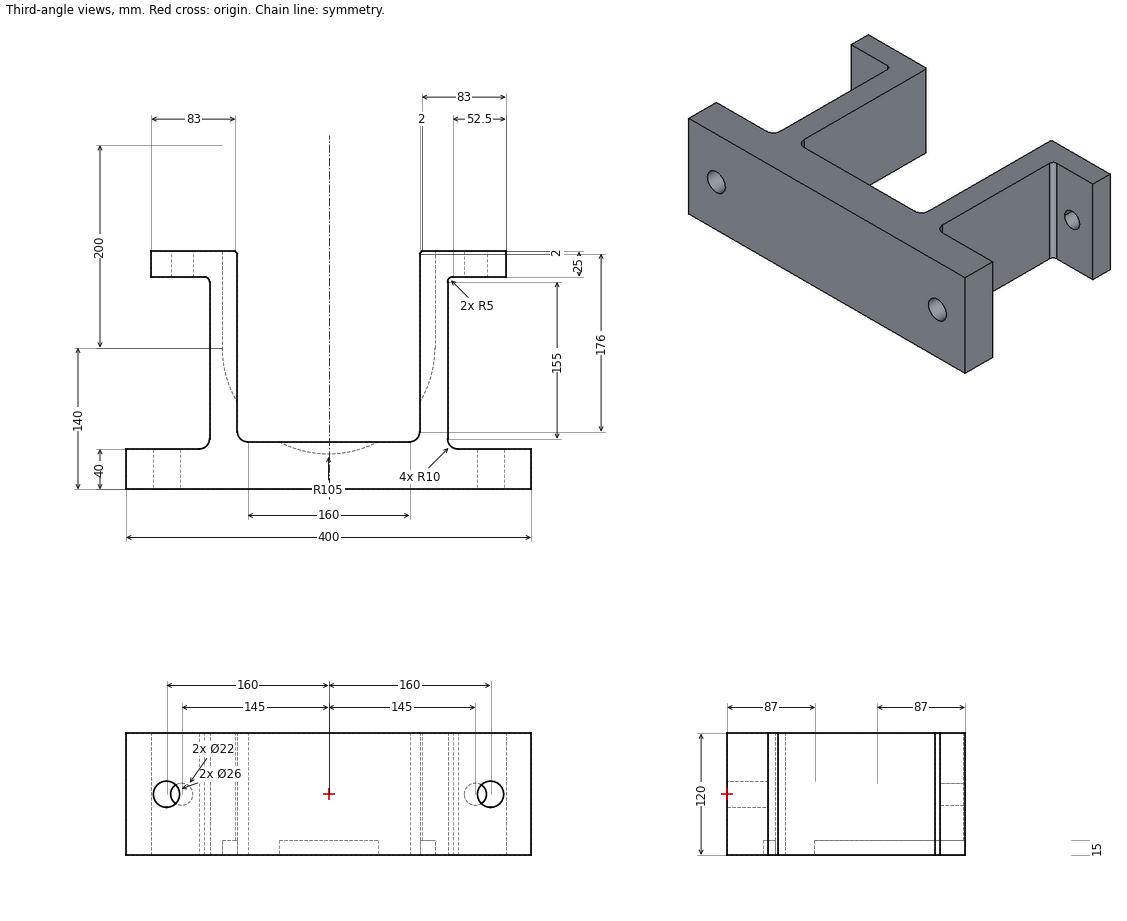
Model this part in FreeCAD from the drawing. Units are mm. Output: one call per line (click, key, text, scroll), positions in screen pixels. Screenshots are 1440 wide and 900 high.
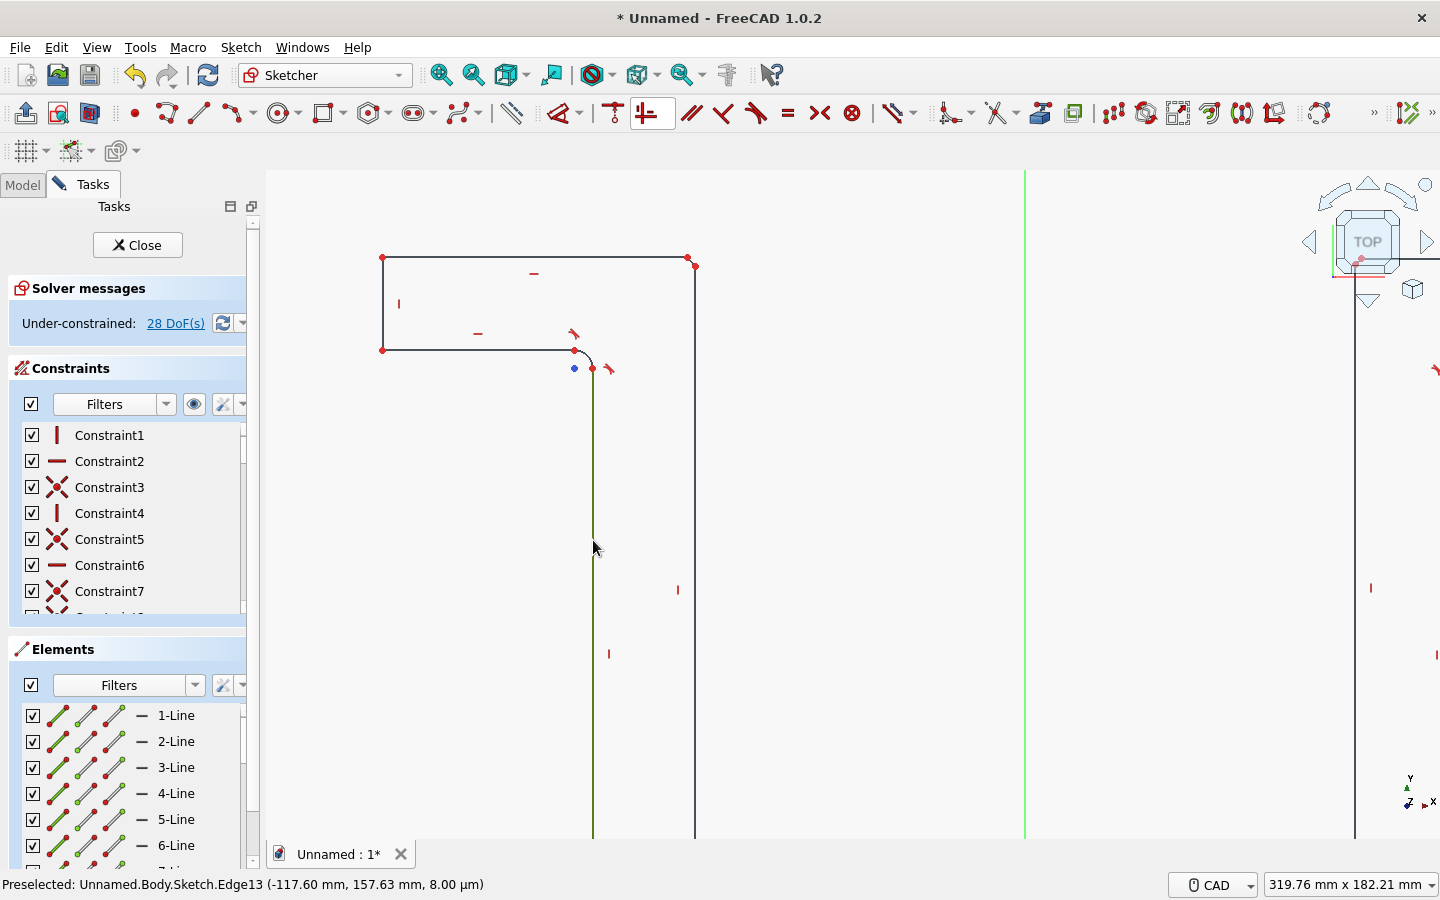
scroll(589, 355, down, 4)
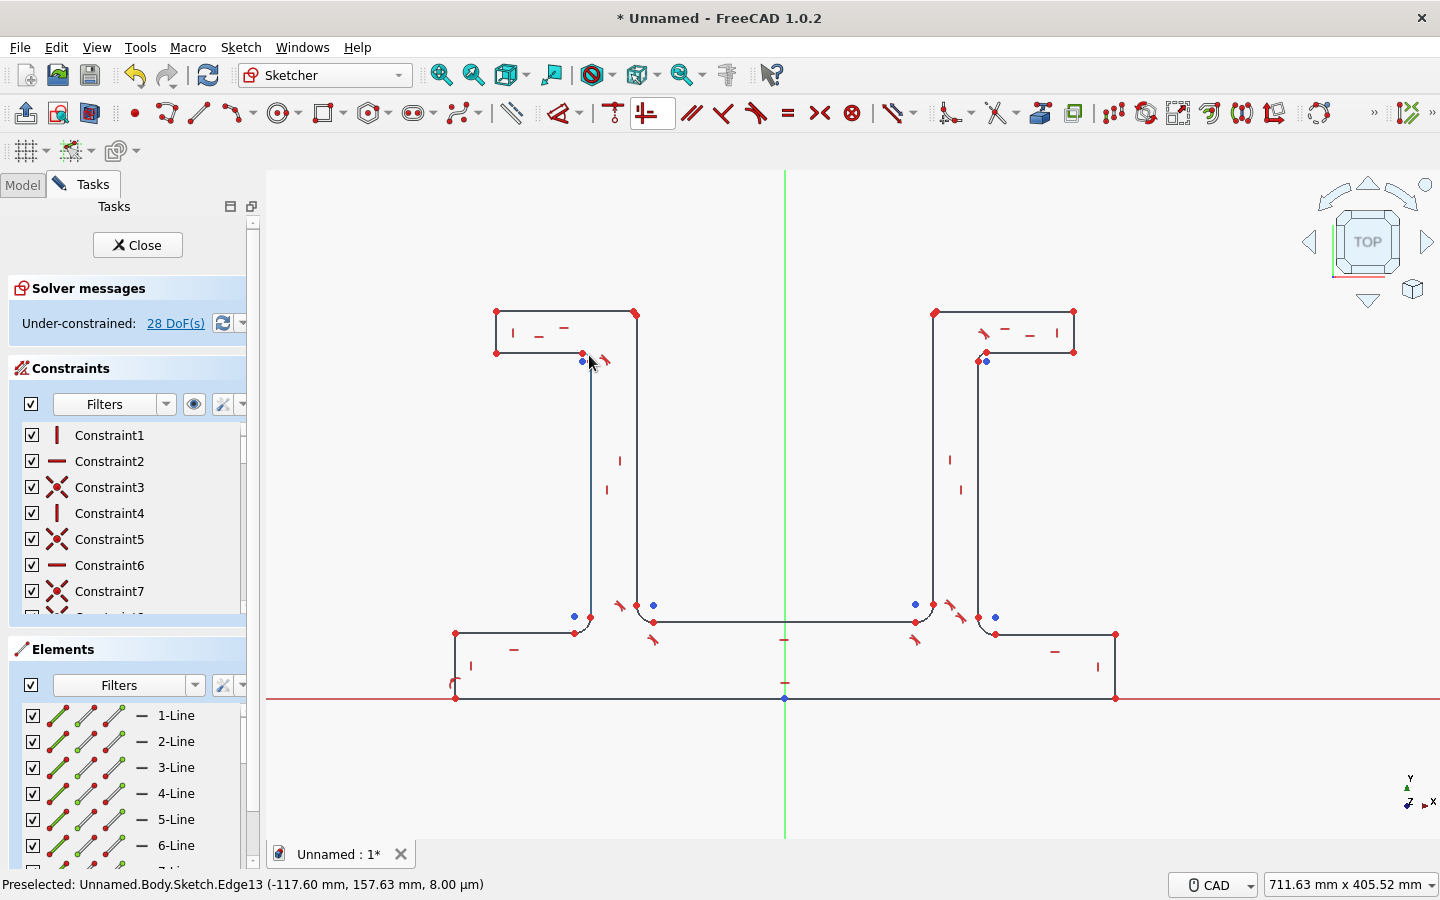
scroll(582, 631, up, 4)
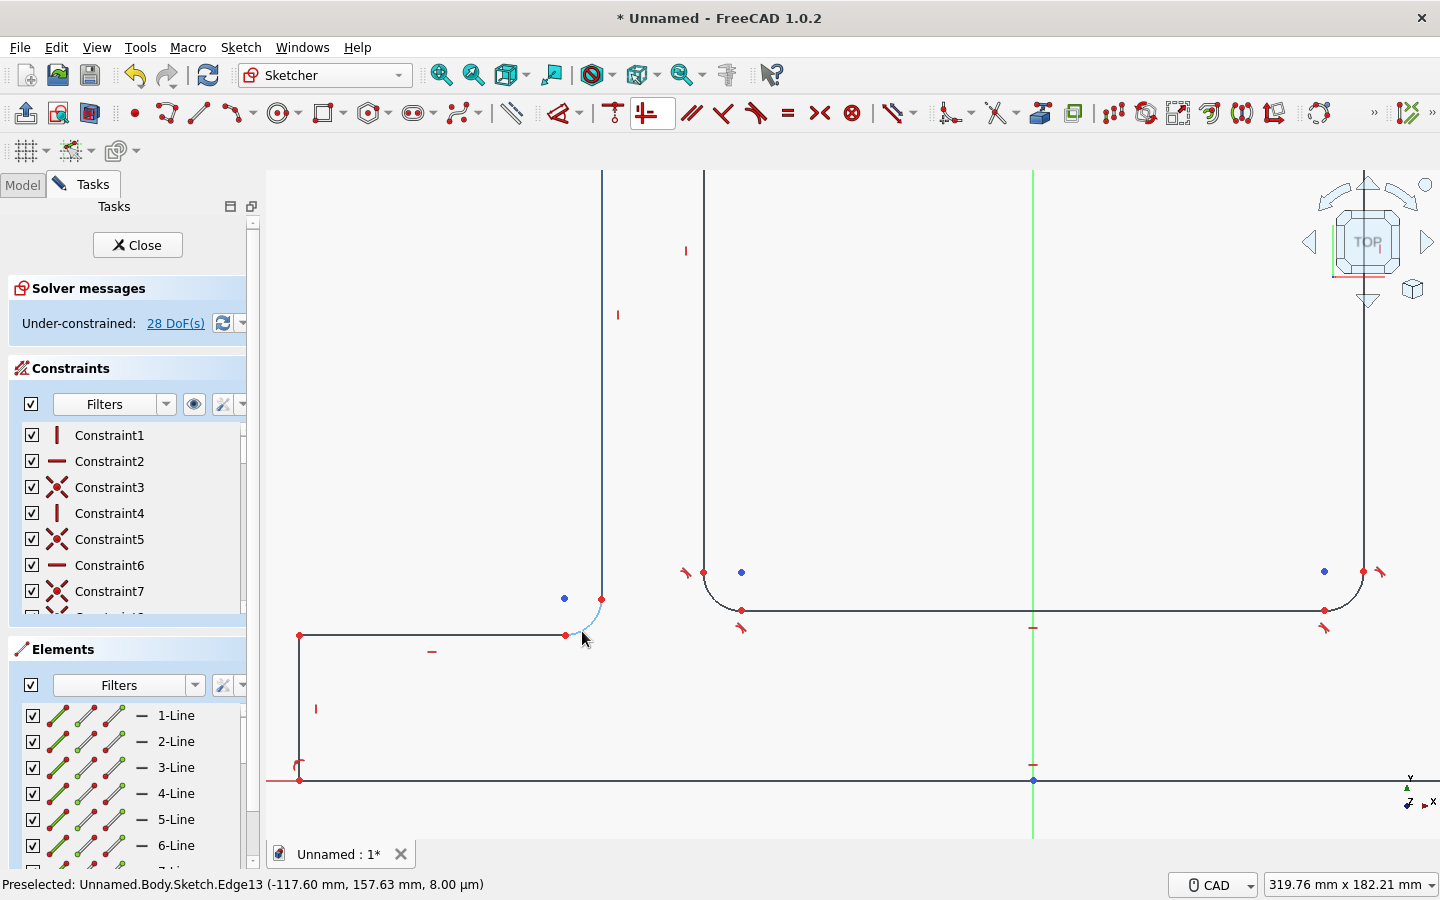
click(582, 631)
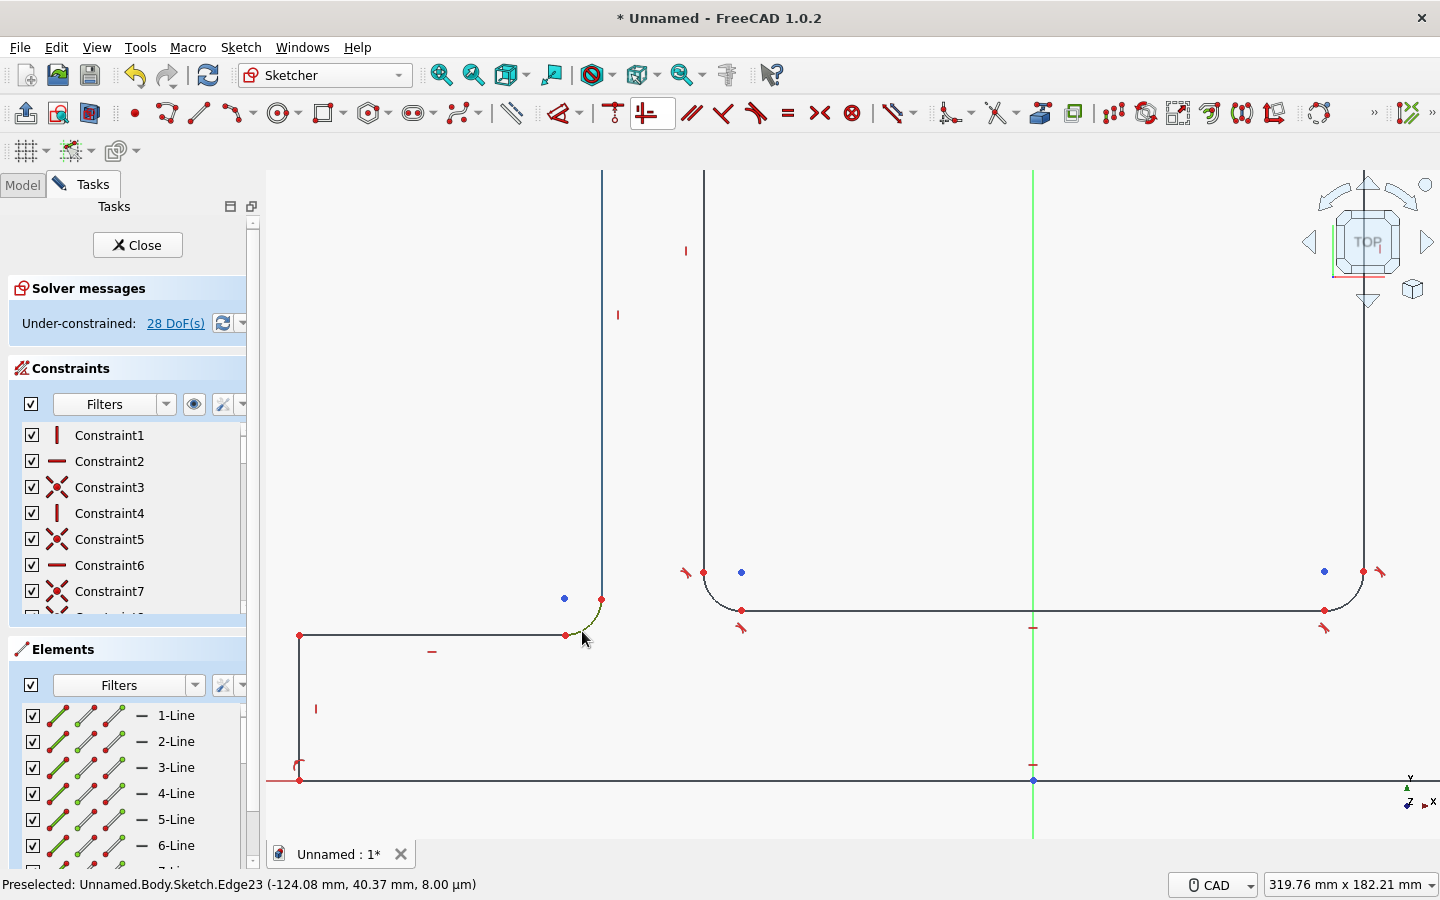
click(756, 114)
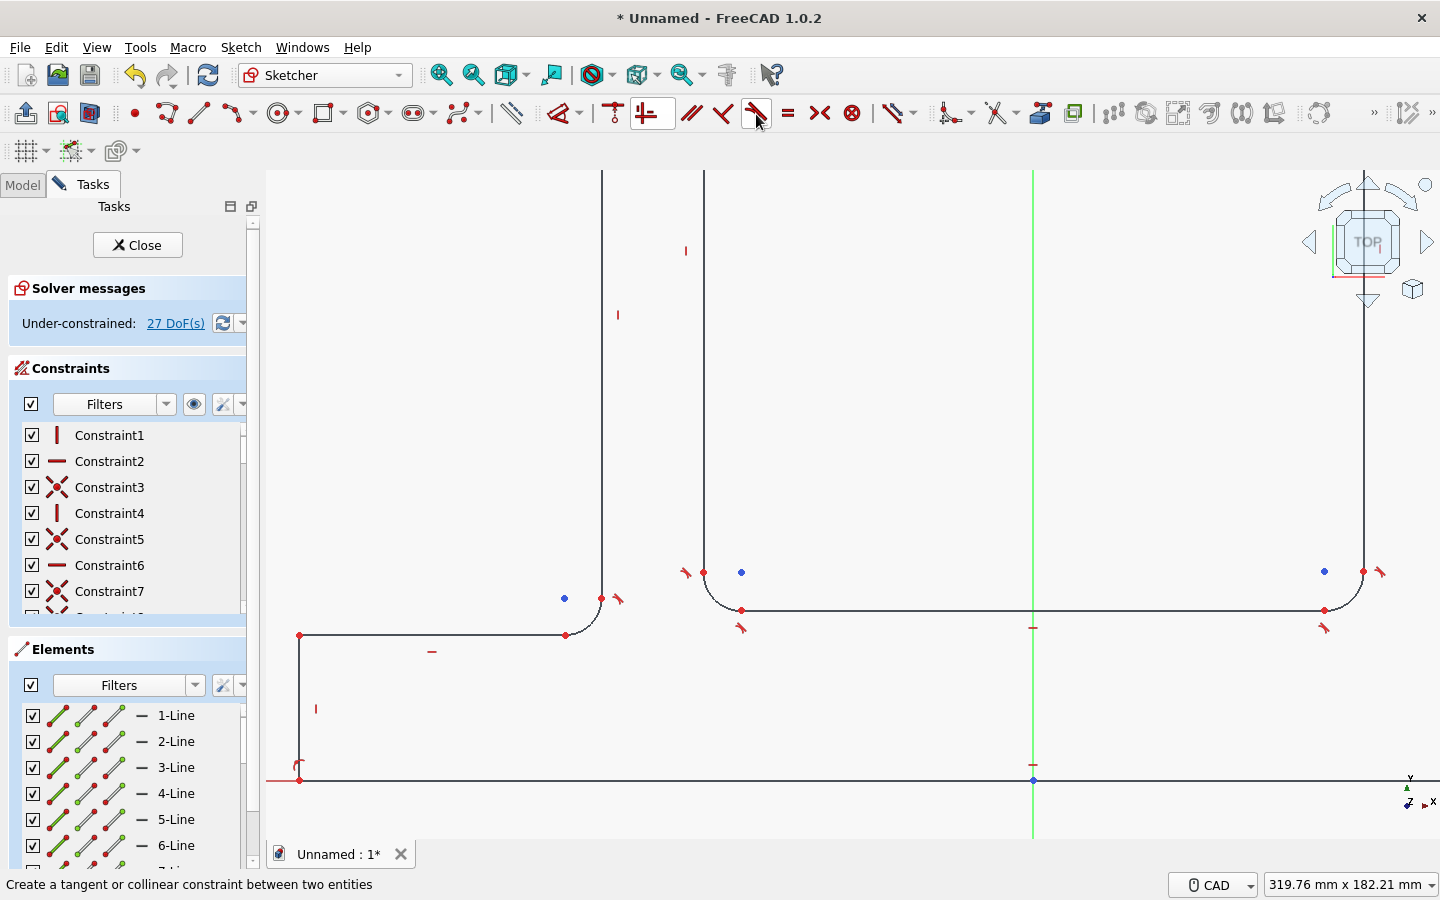
click(486, 635)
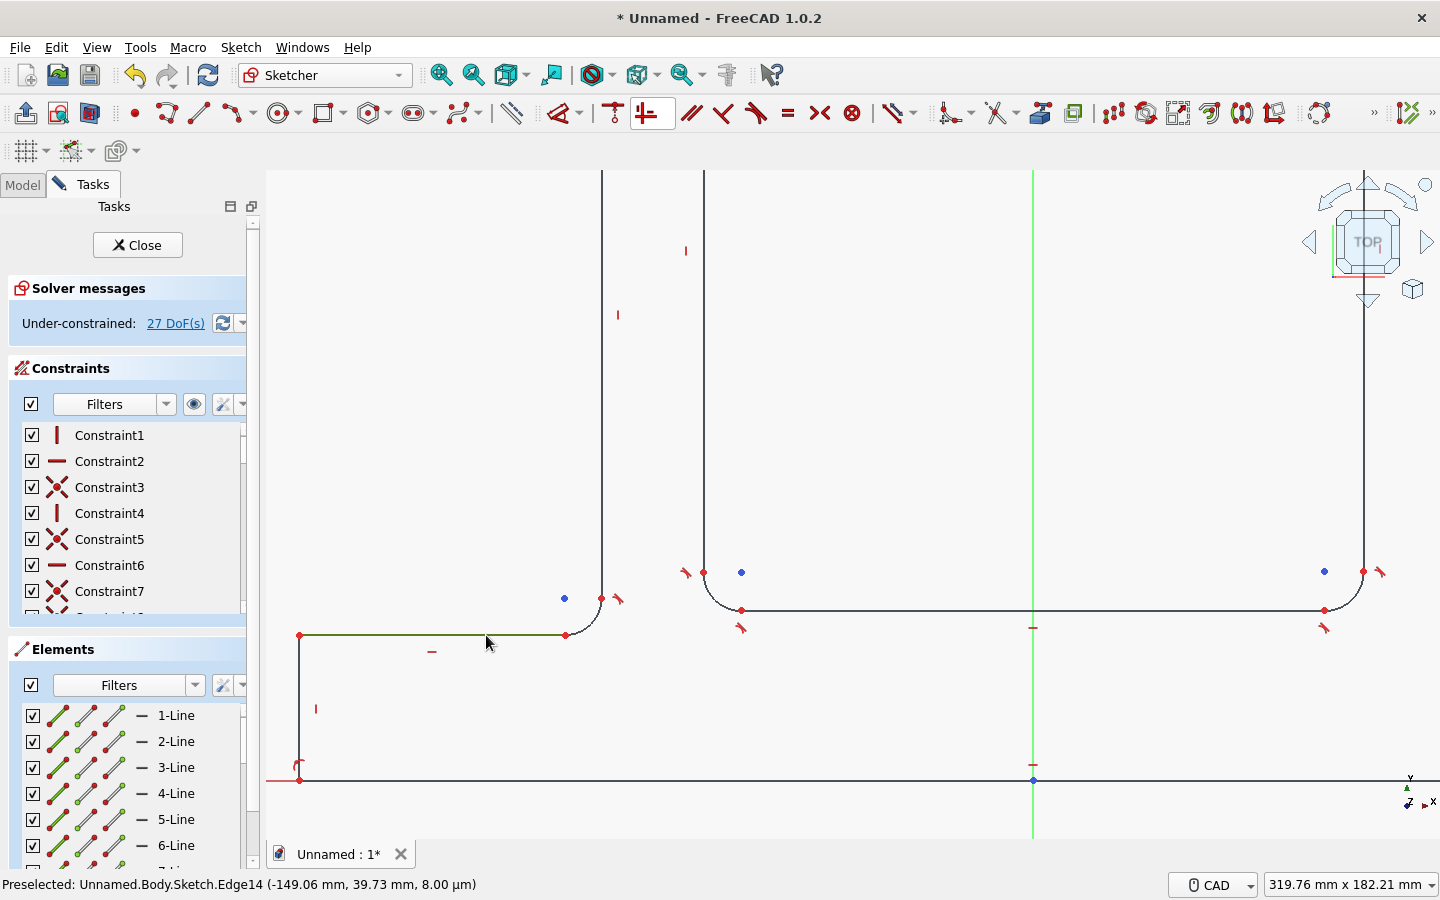
click(582, 631)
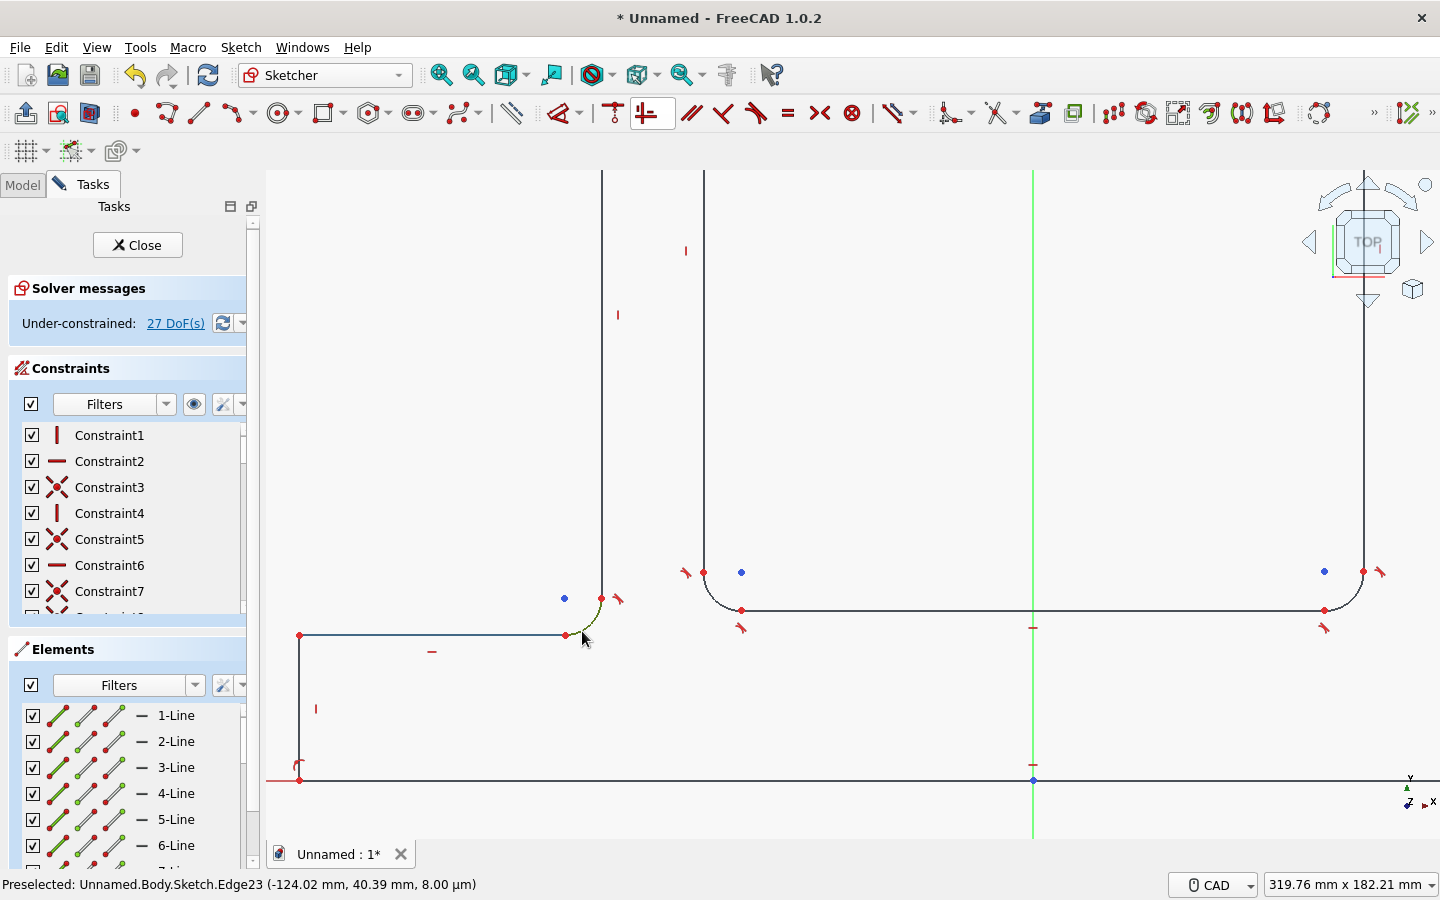
click(756, 114)